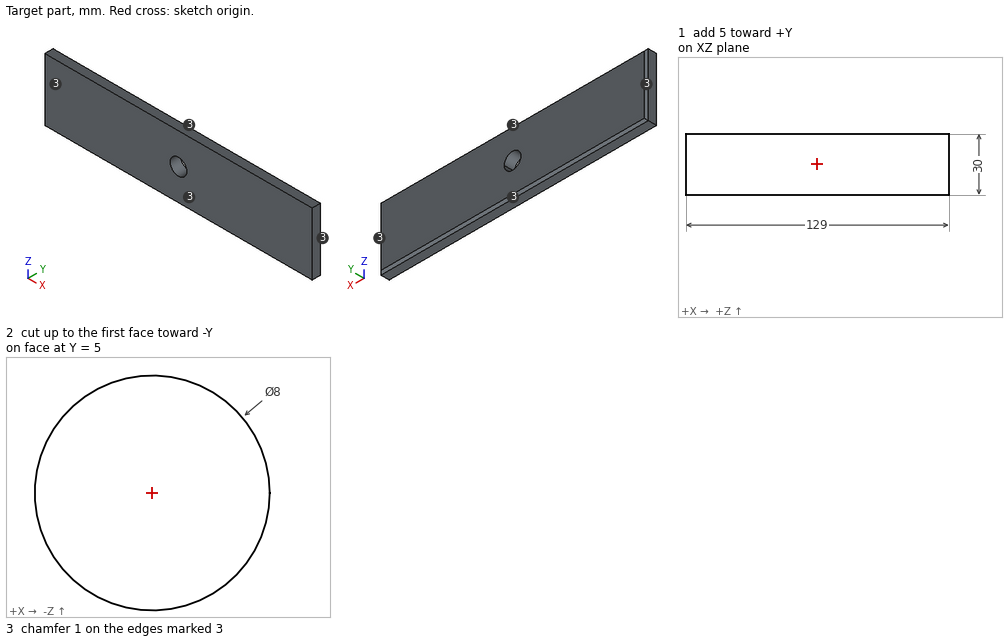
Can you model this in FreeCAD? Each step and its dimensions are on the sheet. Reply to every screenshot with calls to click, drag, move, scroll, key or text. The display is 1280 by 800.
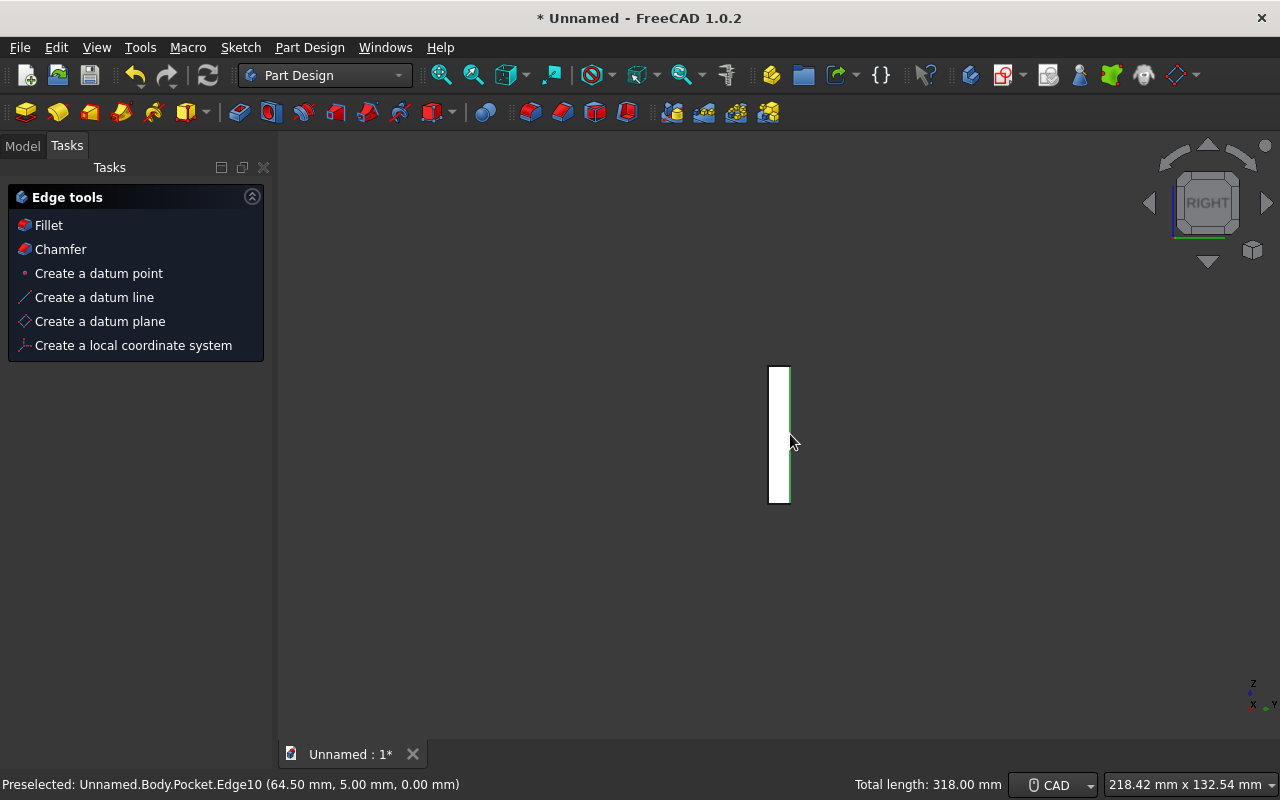
click(564, 112)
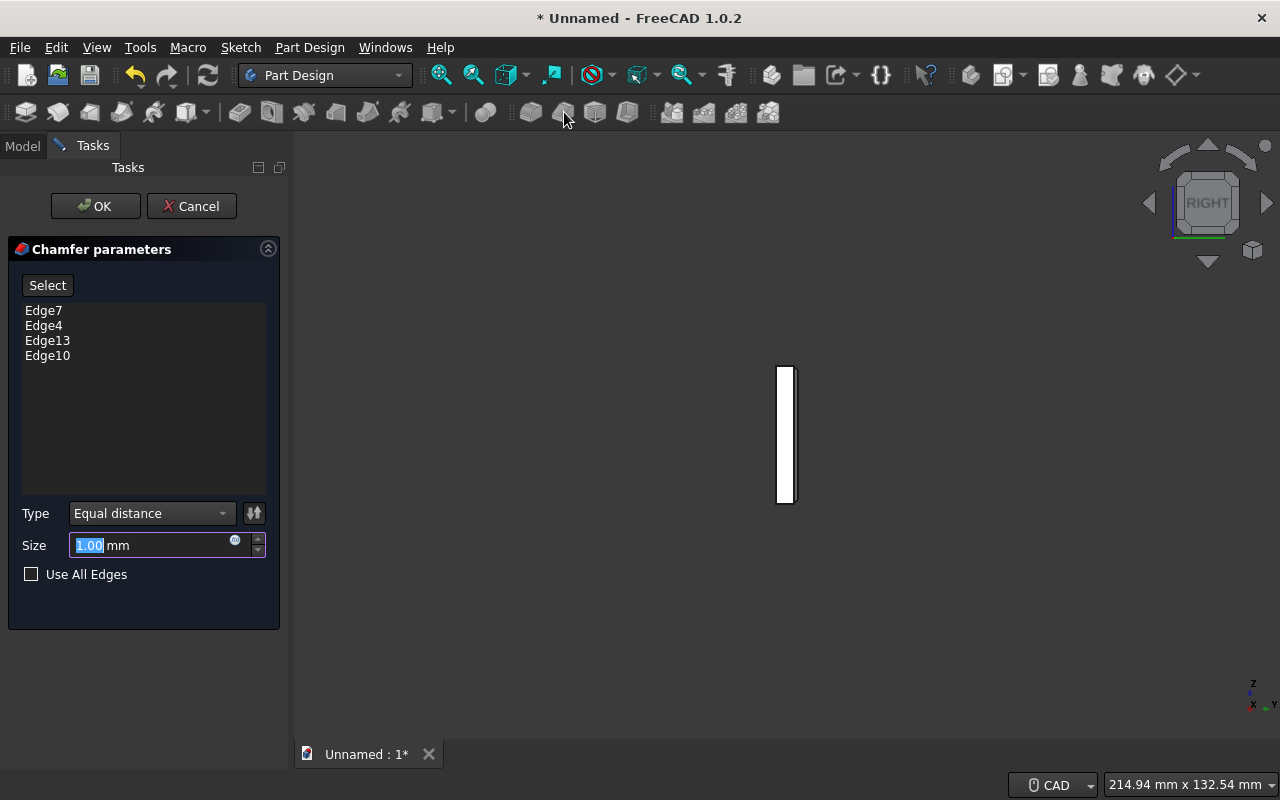
text(1)
key(Tab)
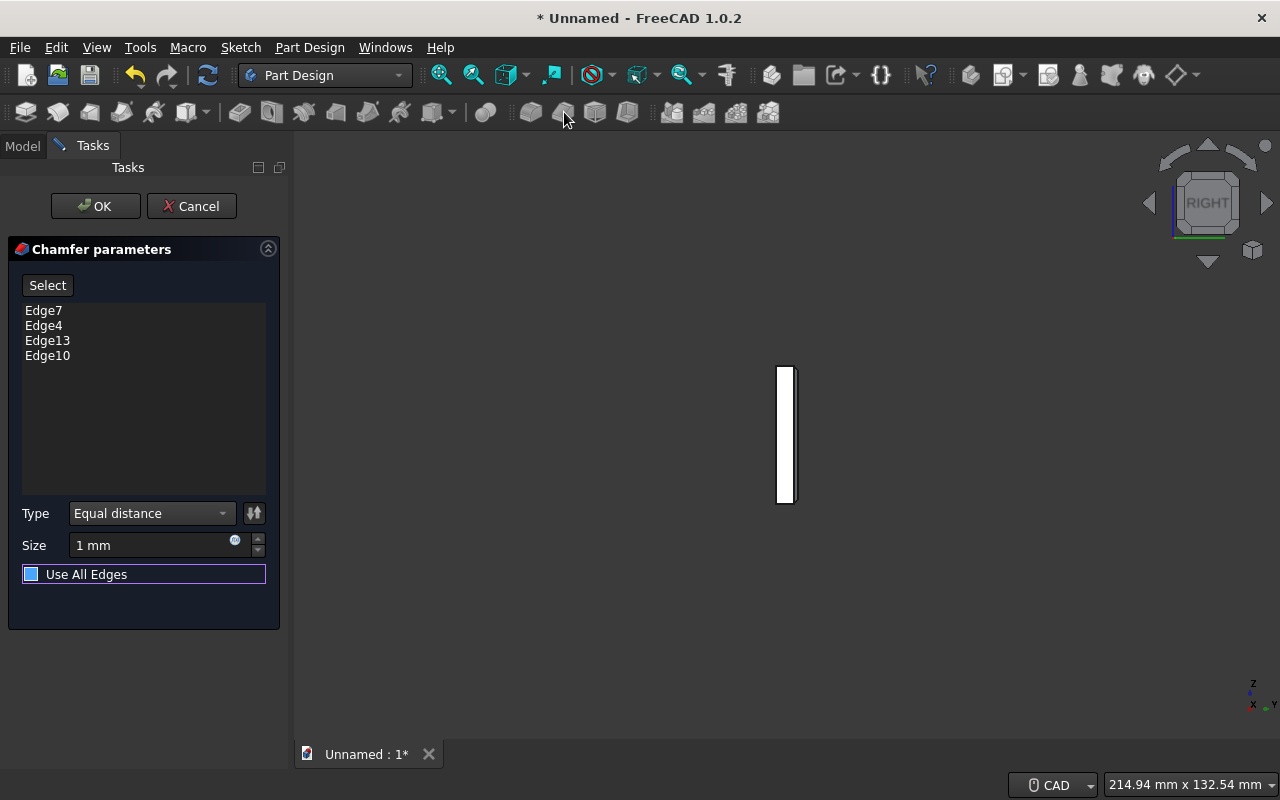
click(96, 206)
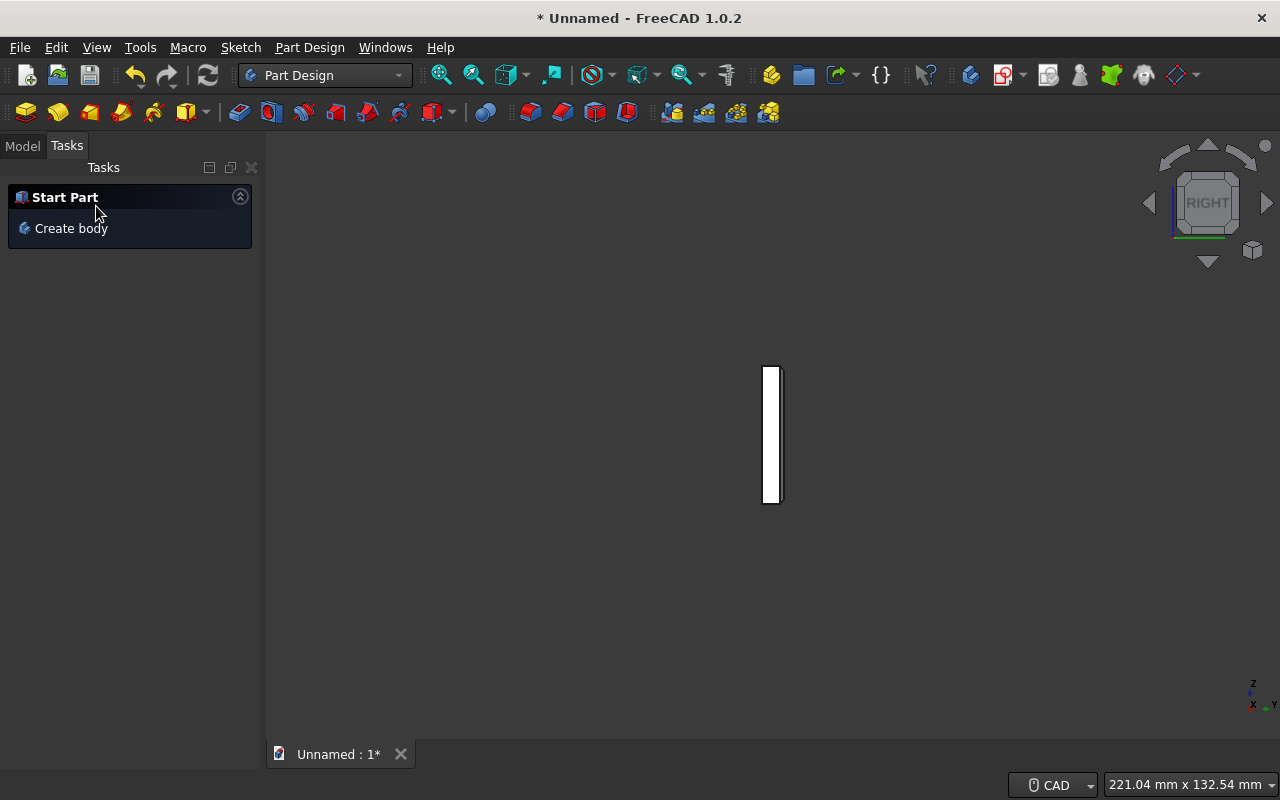
key(0)